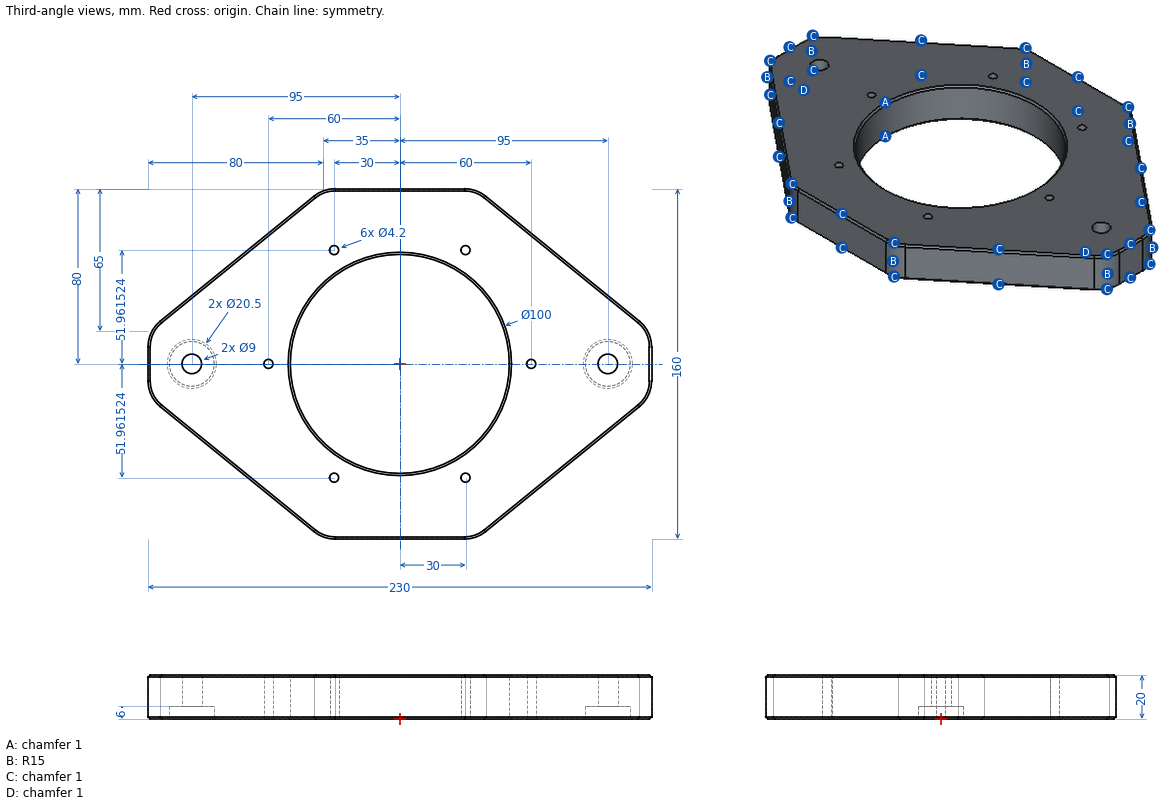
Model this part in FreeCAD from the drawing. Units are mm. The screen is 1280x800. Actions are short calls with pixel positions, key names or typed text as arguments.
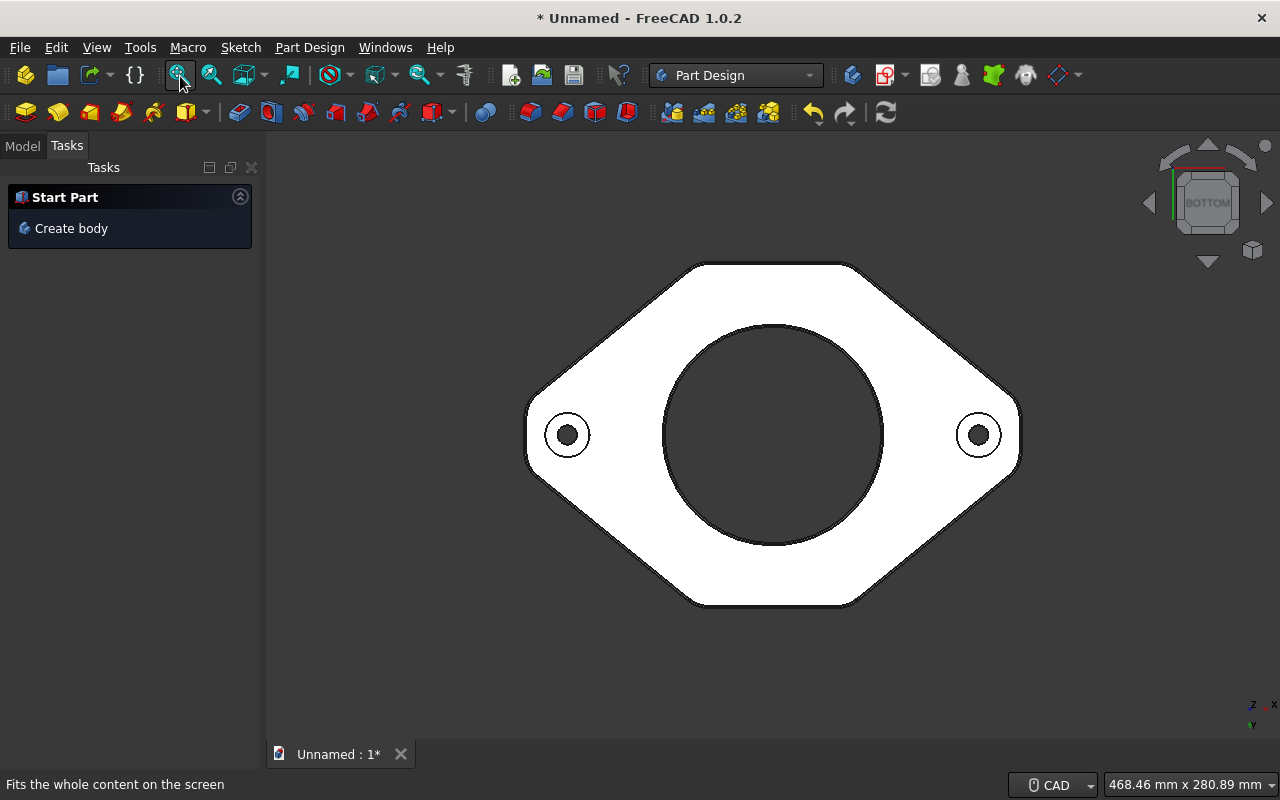
click(545, 434)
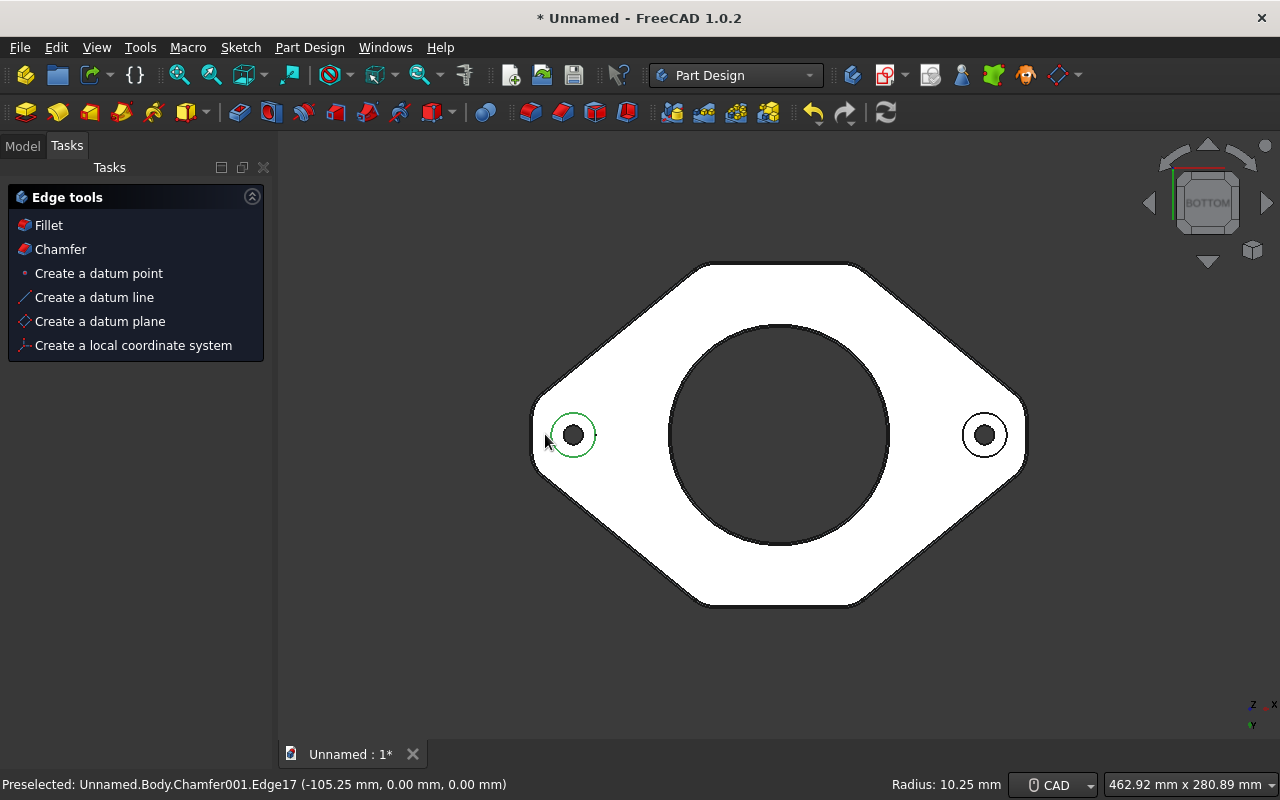
click(962, 434, ctrl)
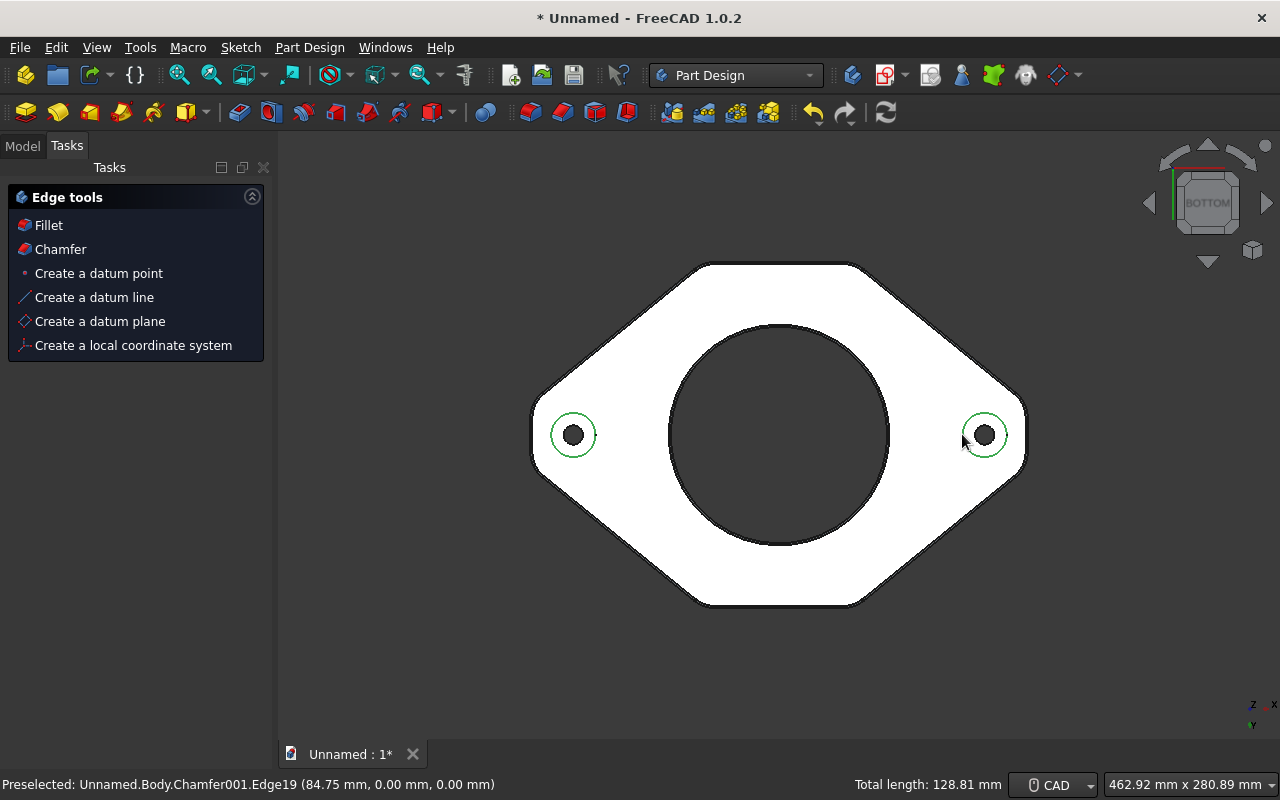
click(564, 112)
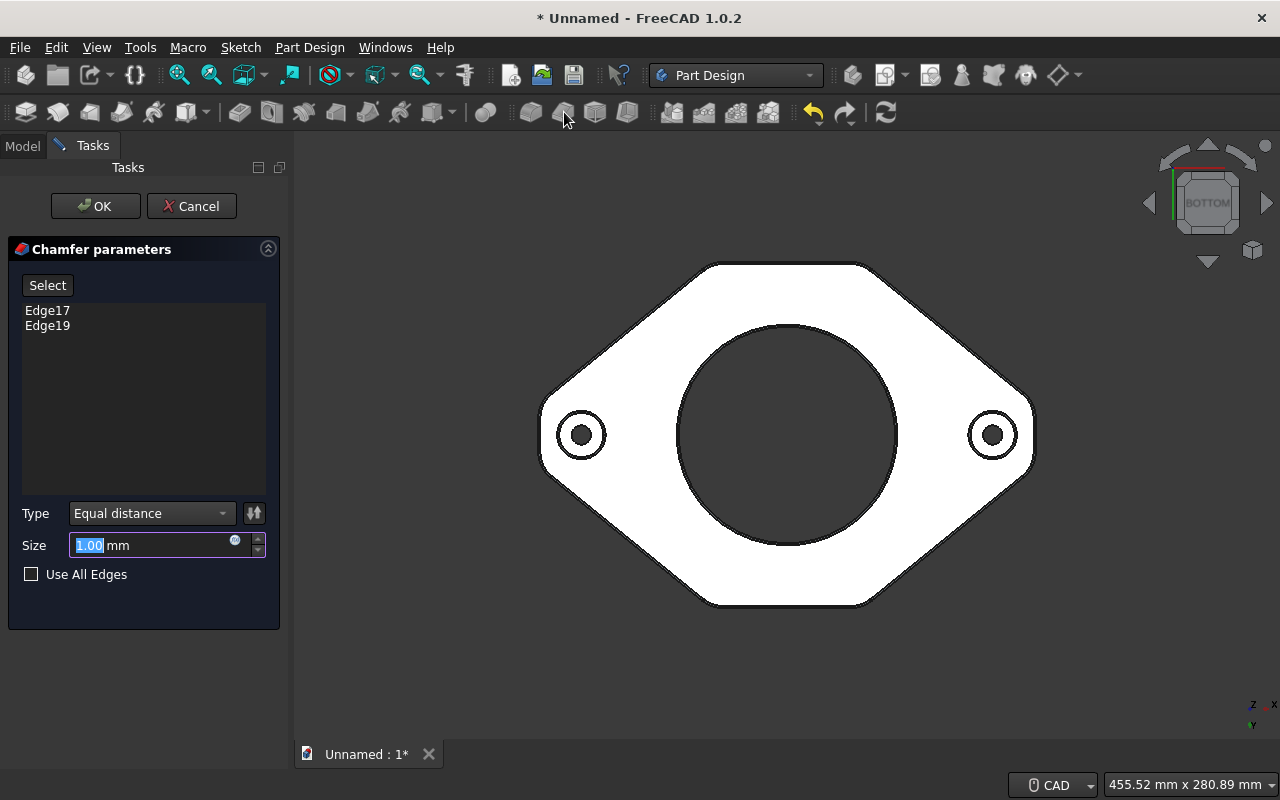
text(1)
key(Tab)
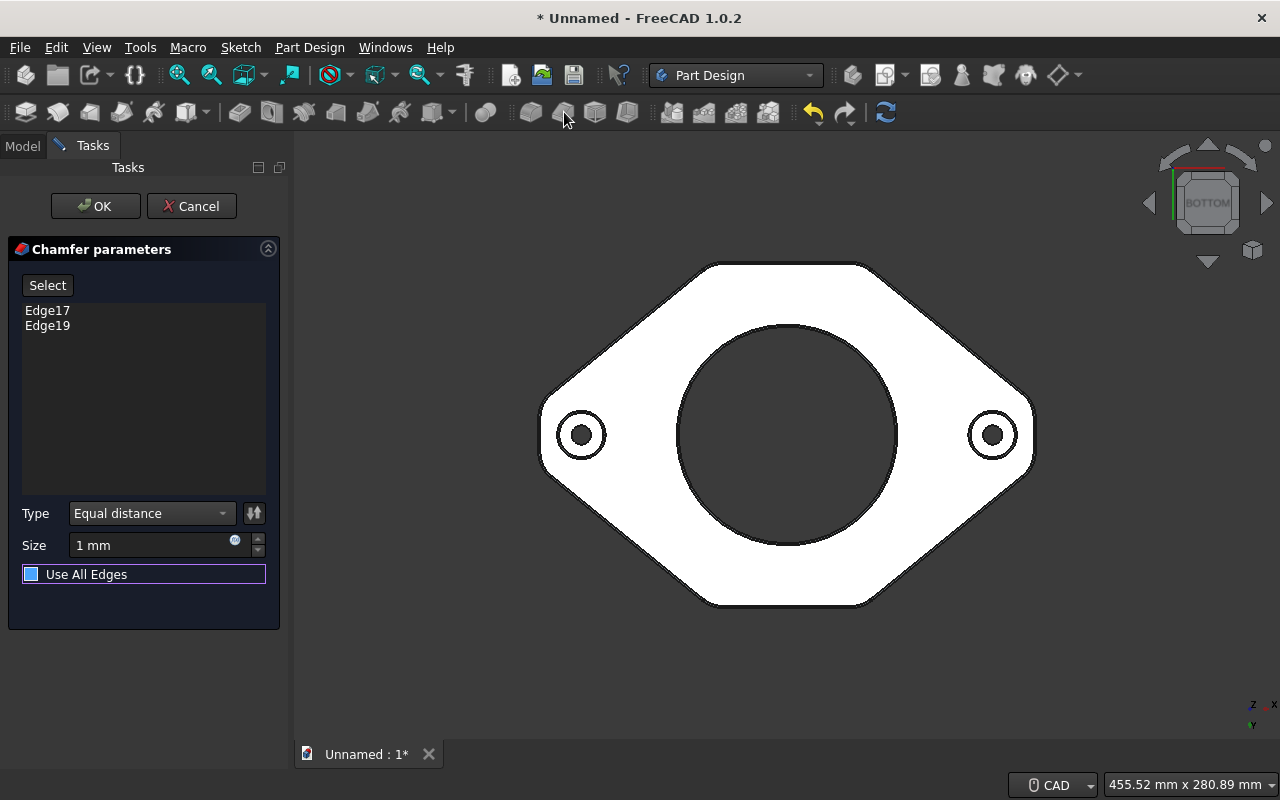
click(96, 206)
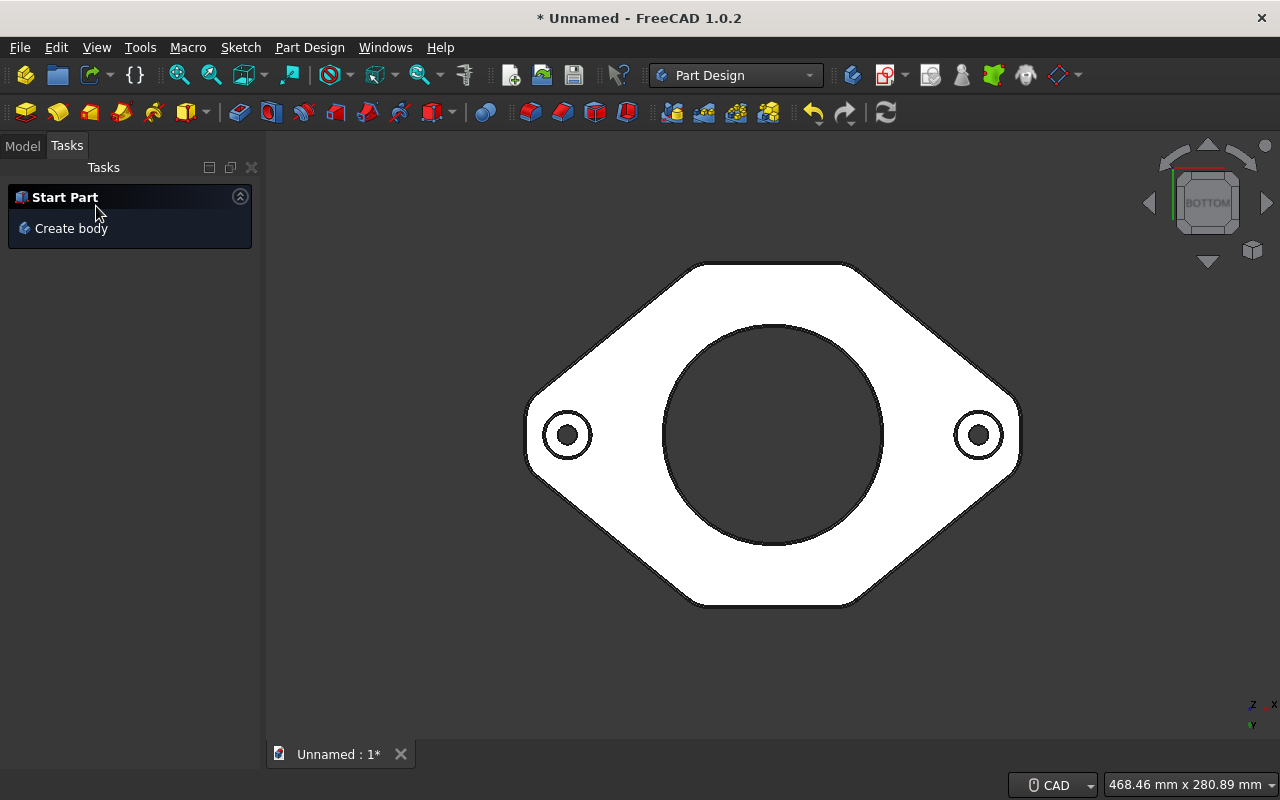
key(0)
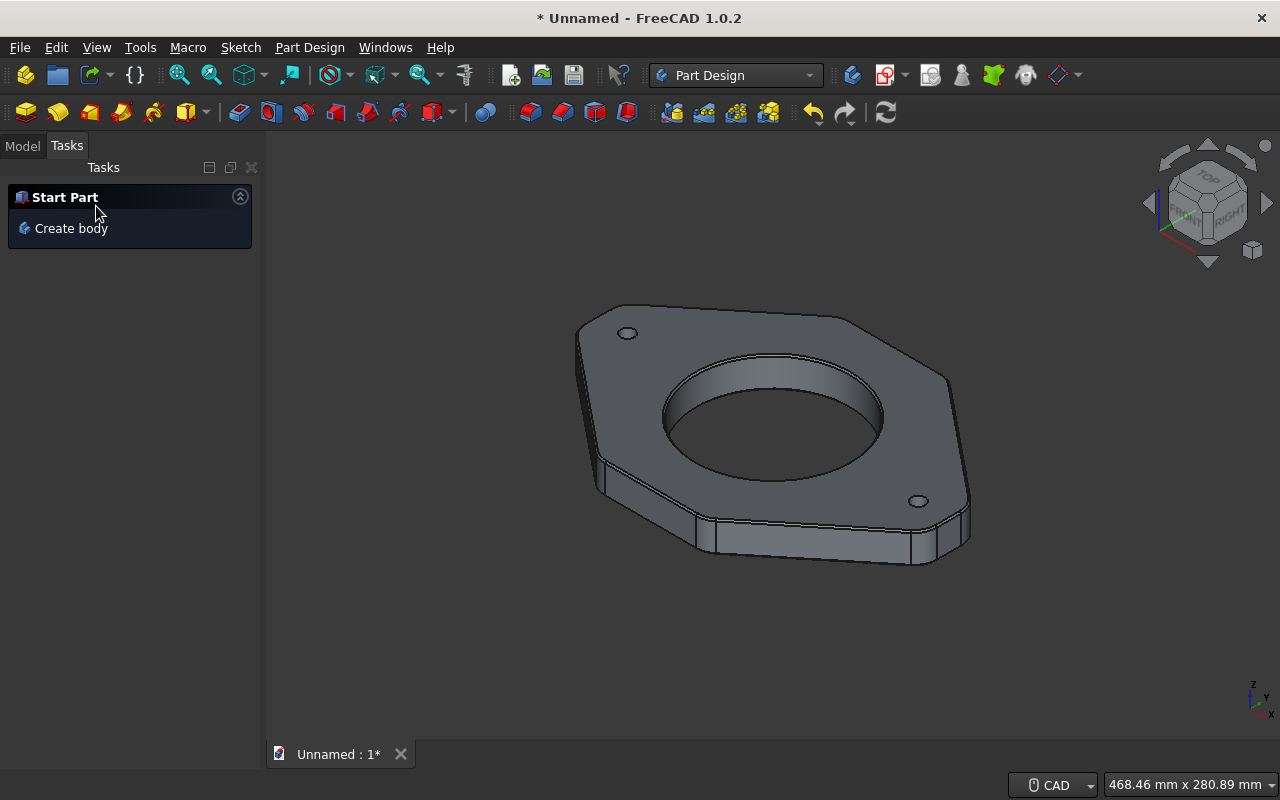
click(907, 454)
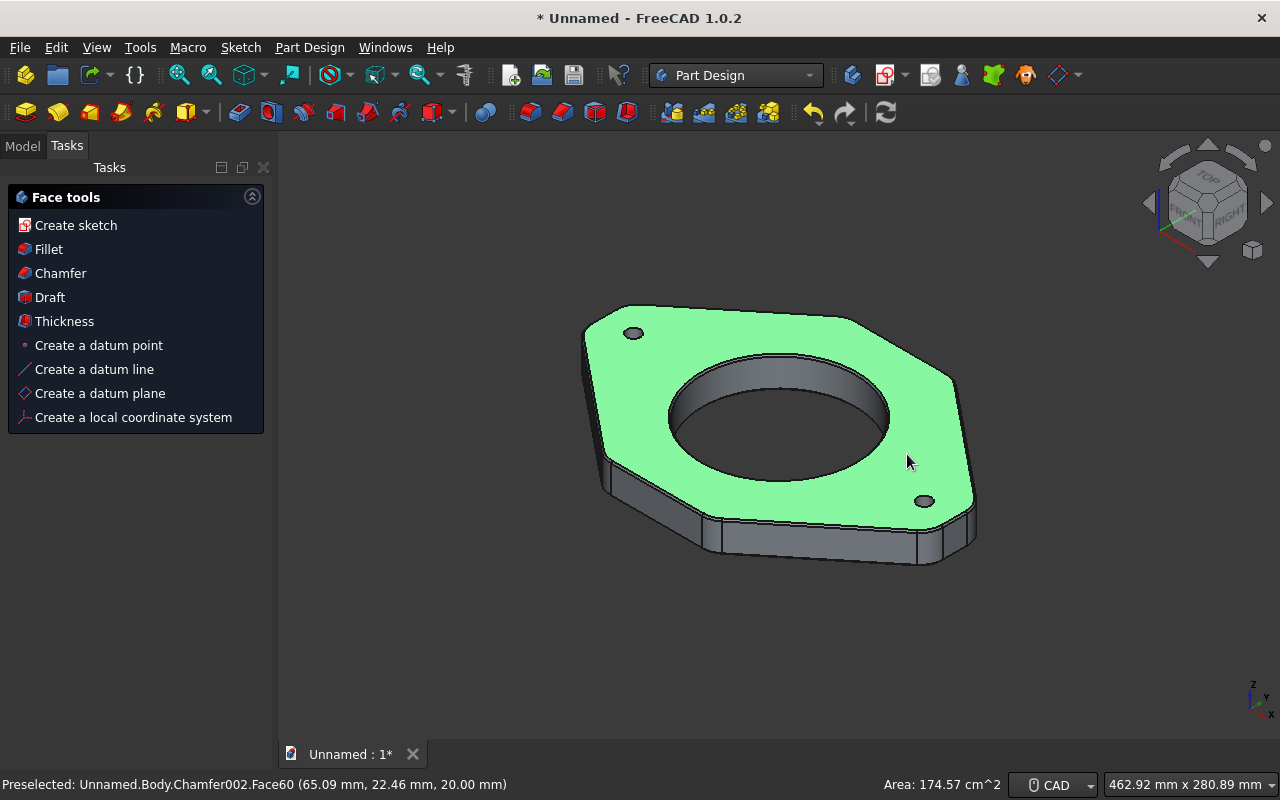
click(886, 76)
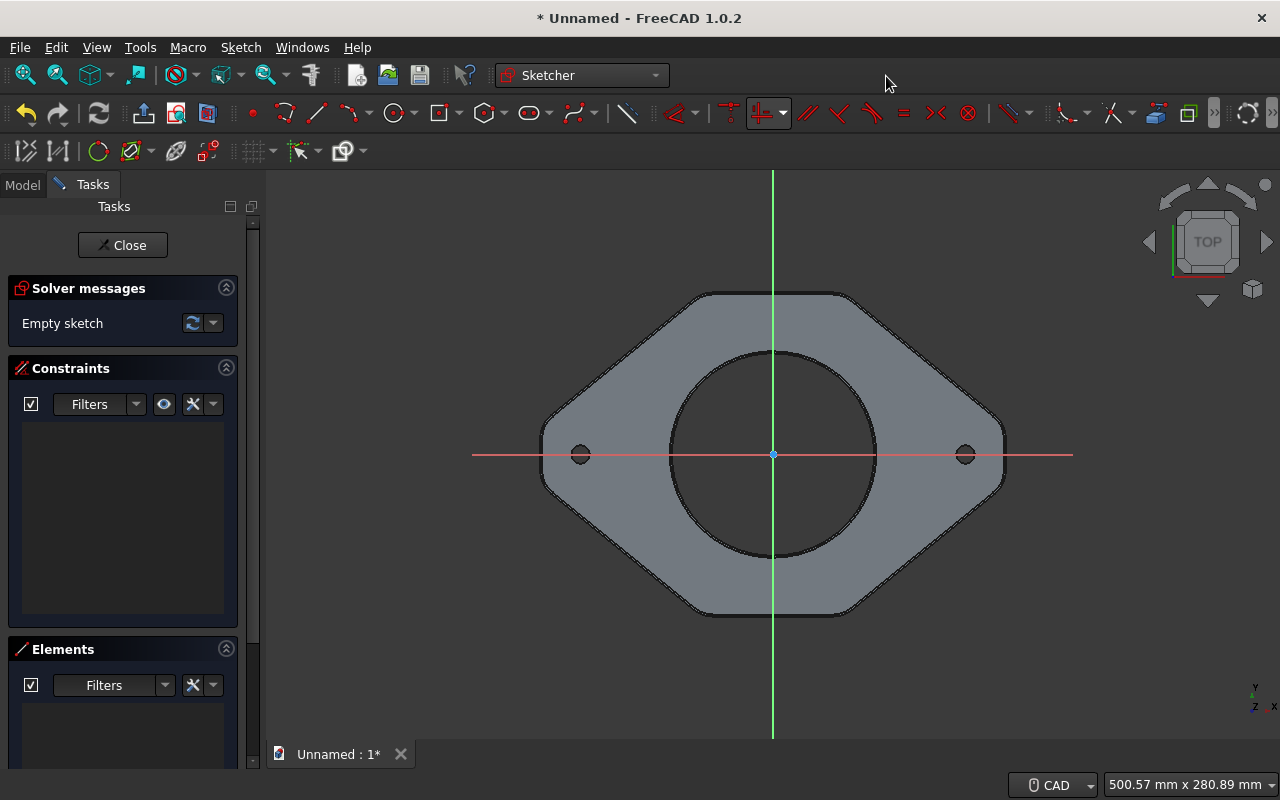
scroll(856, 454, up, 3)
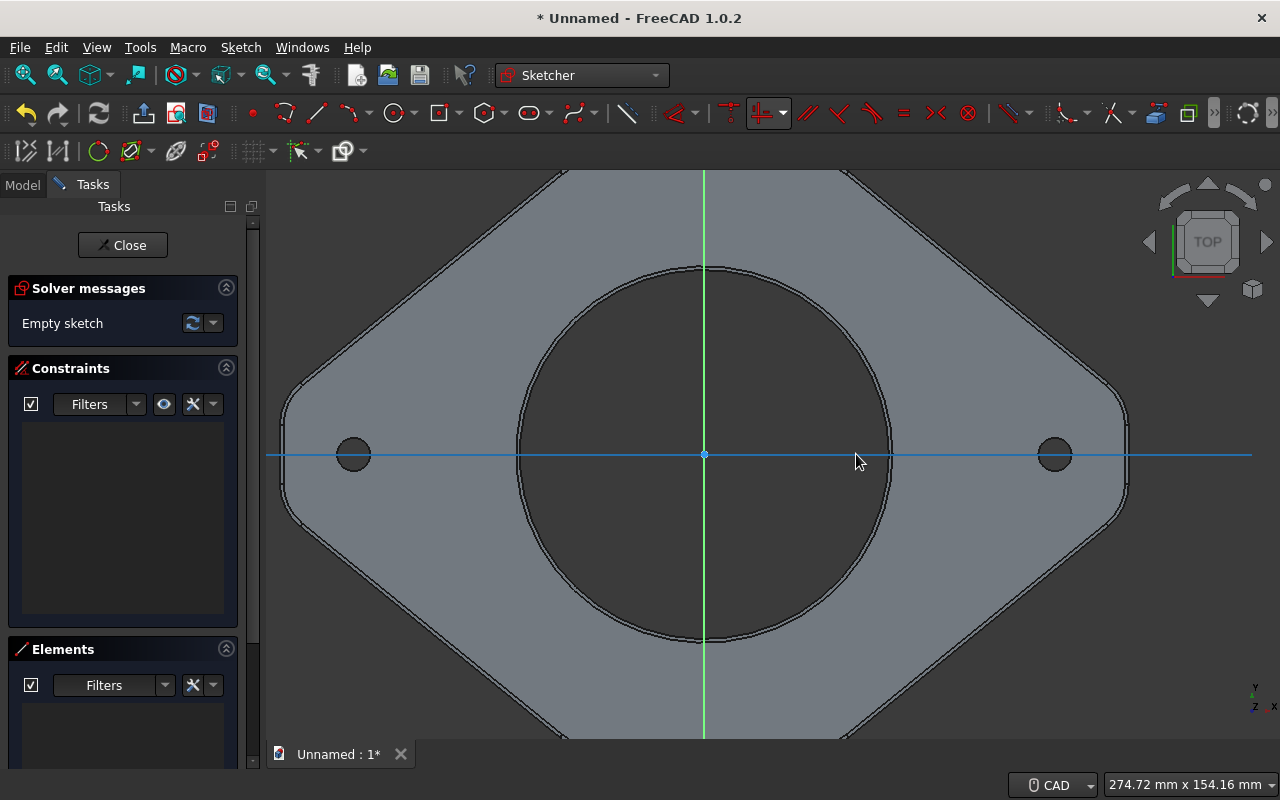
click(394, 114)